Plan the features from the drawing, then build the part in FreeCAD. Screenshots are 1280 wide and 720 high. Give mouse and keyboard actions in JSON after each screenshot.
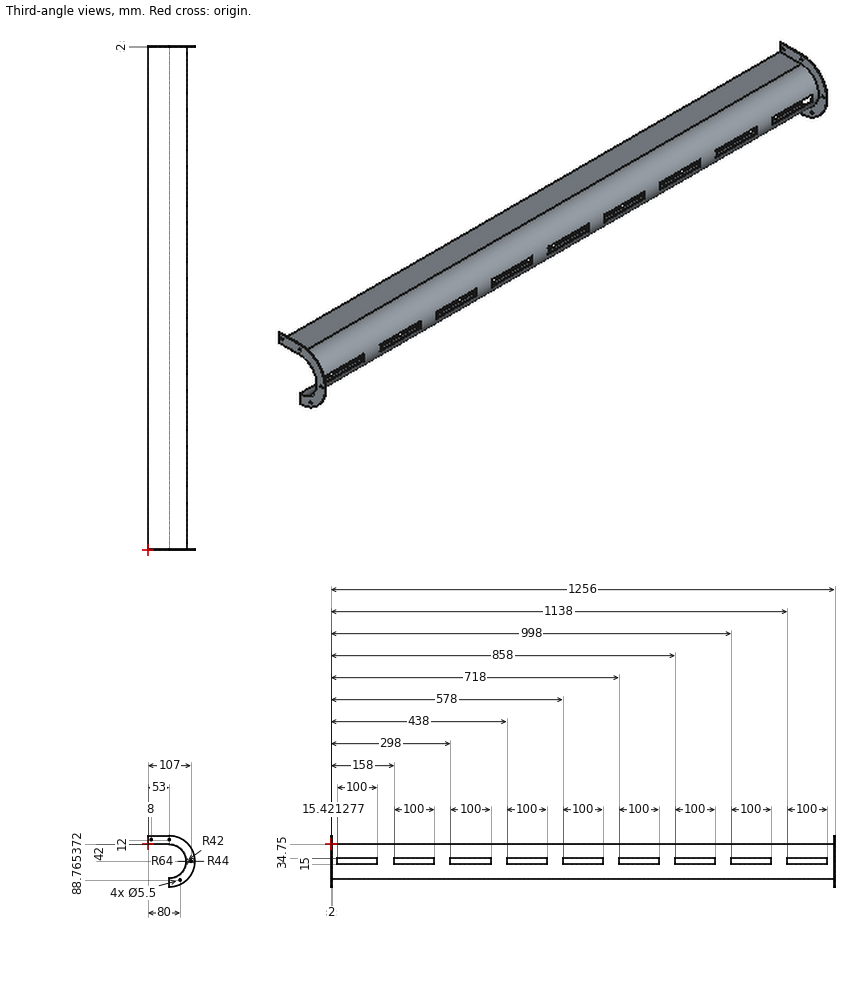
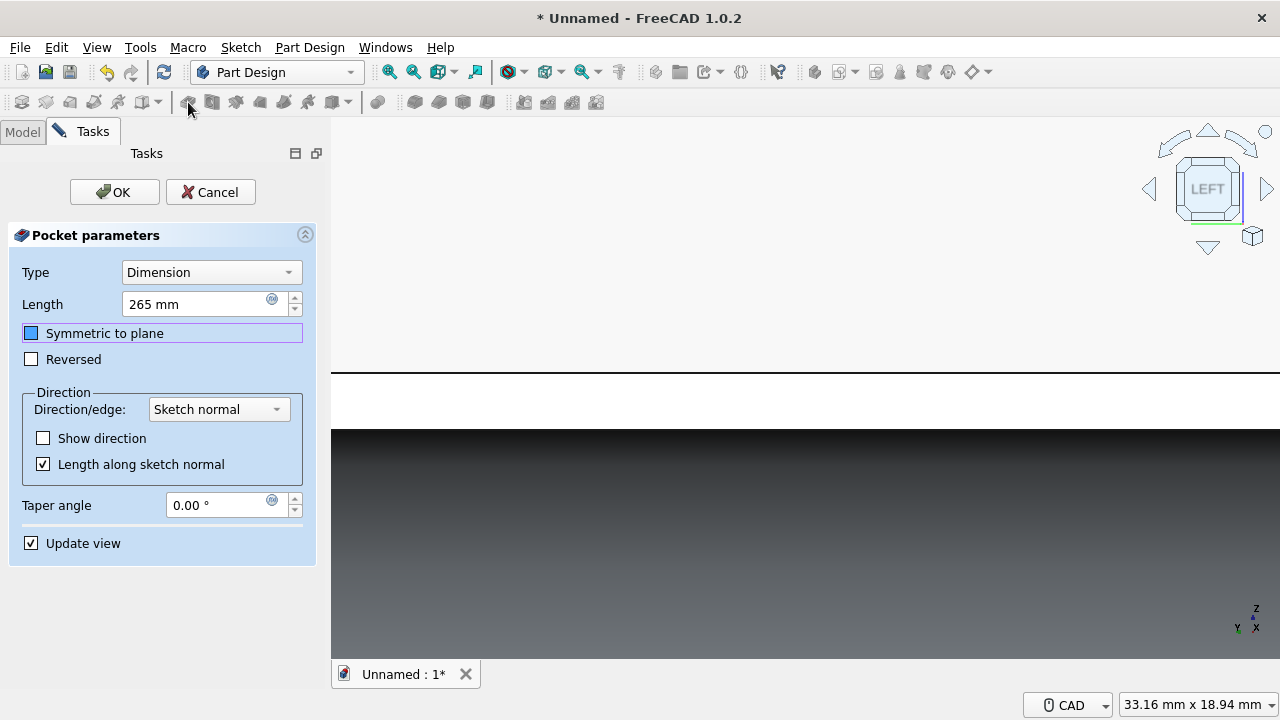
{"action": "left_click", "coordinate": [115, 192]}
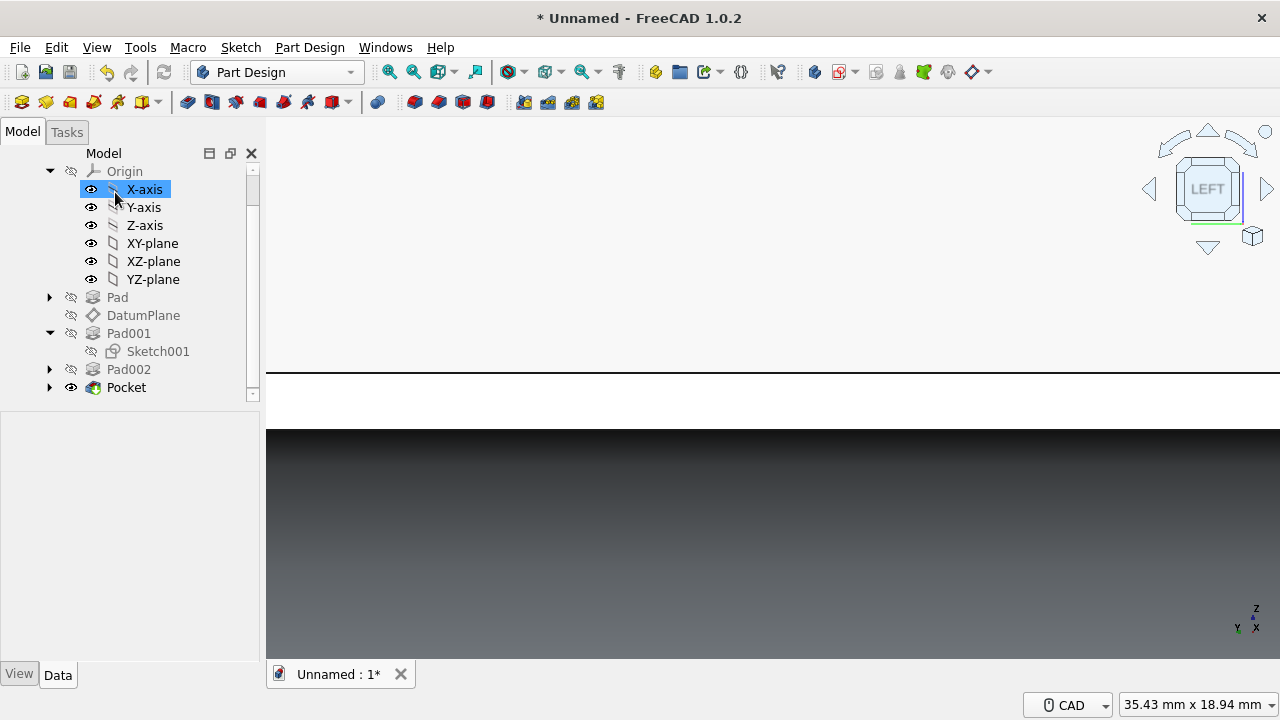
{"action": "left_click", "coordinate": [390, 72]}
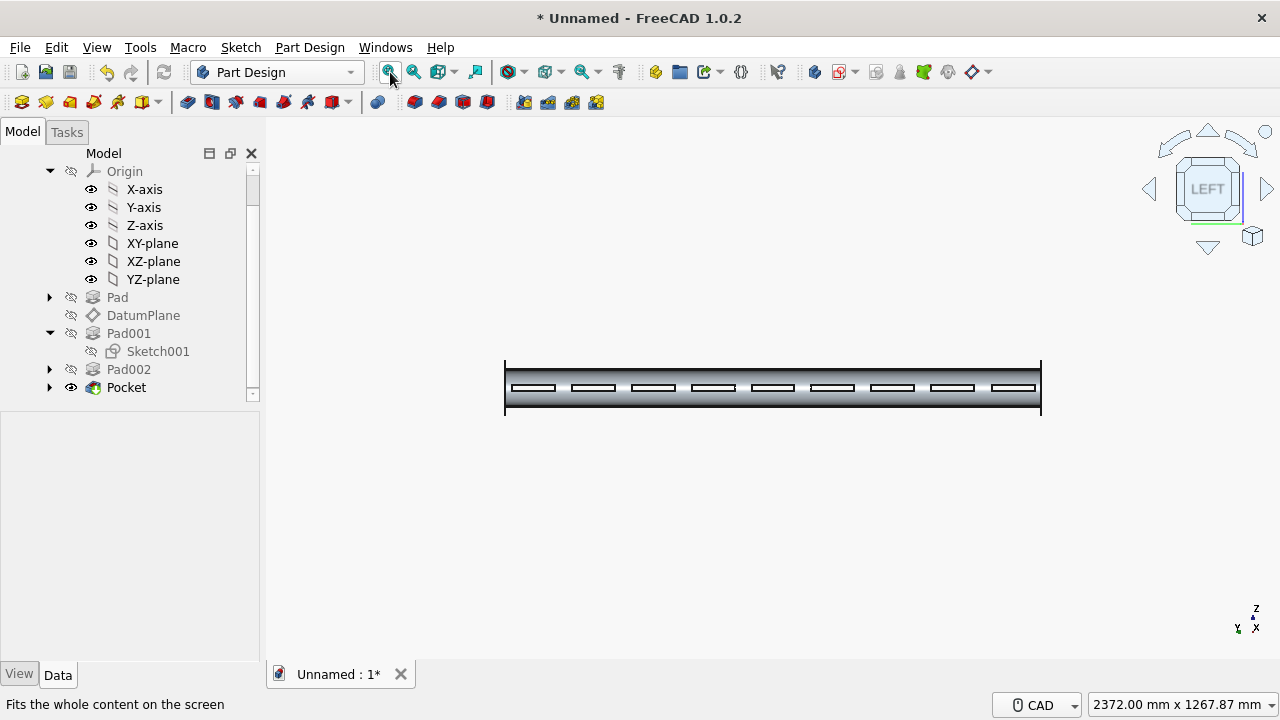
{"action": "key", "text": "4"}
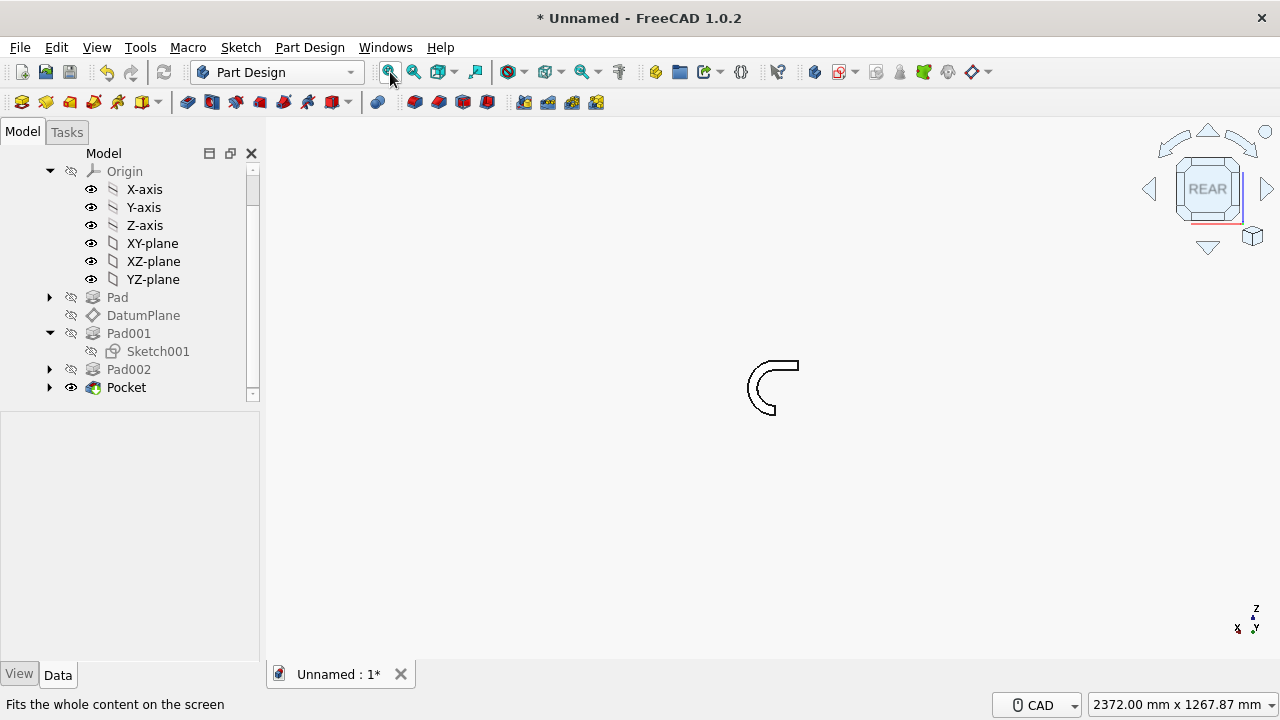
{"action": "left_click", "coordinate": [390, 72]}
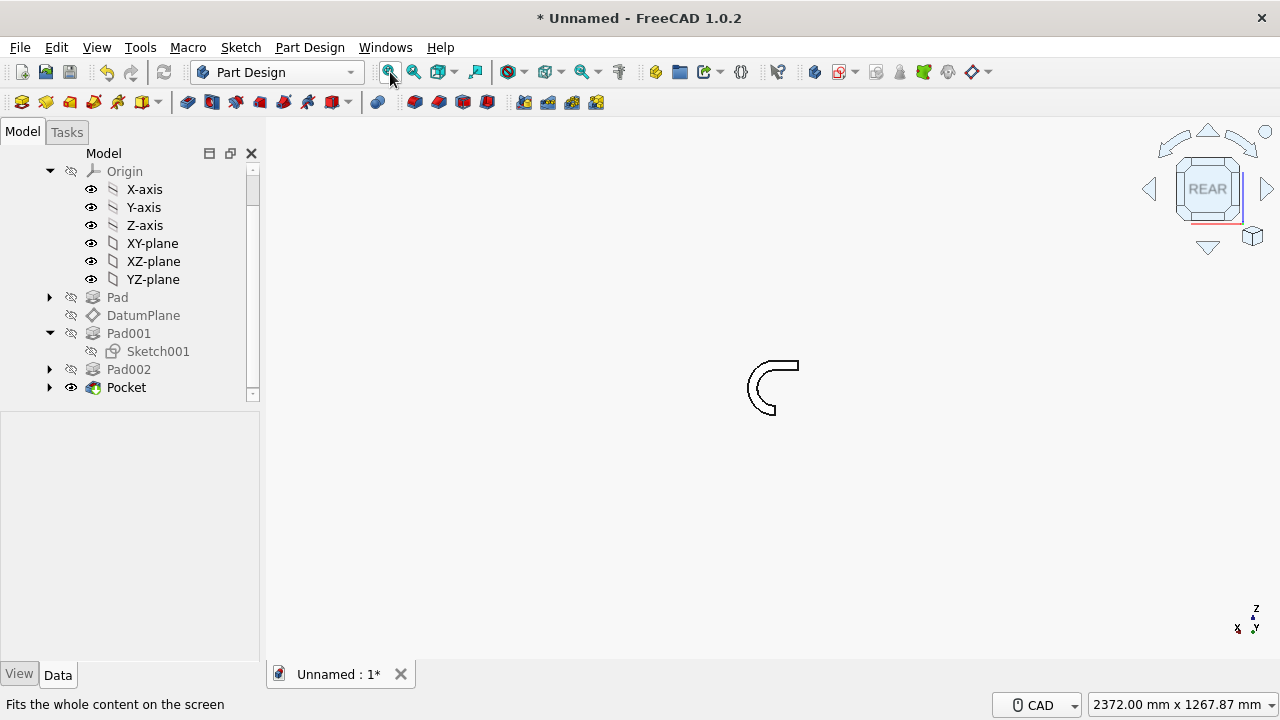
{"action": "scroll", "coordinate": [759, 403], "scroll_direction": "up", "scroll_amount": 5}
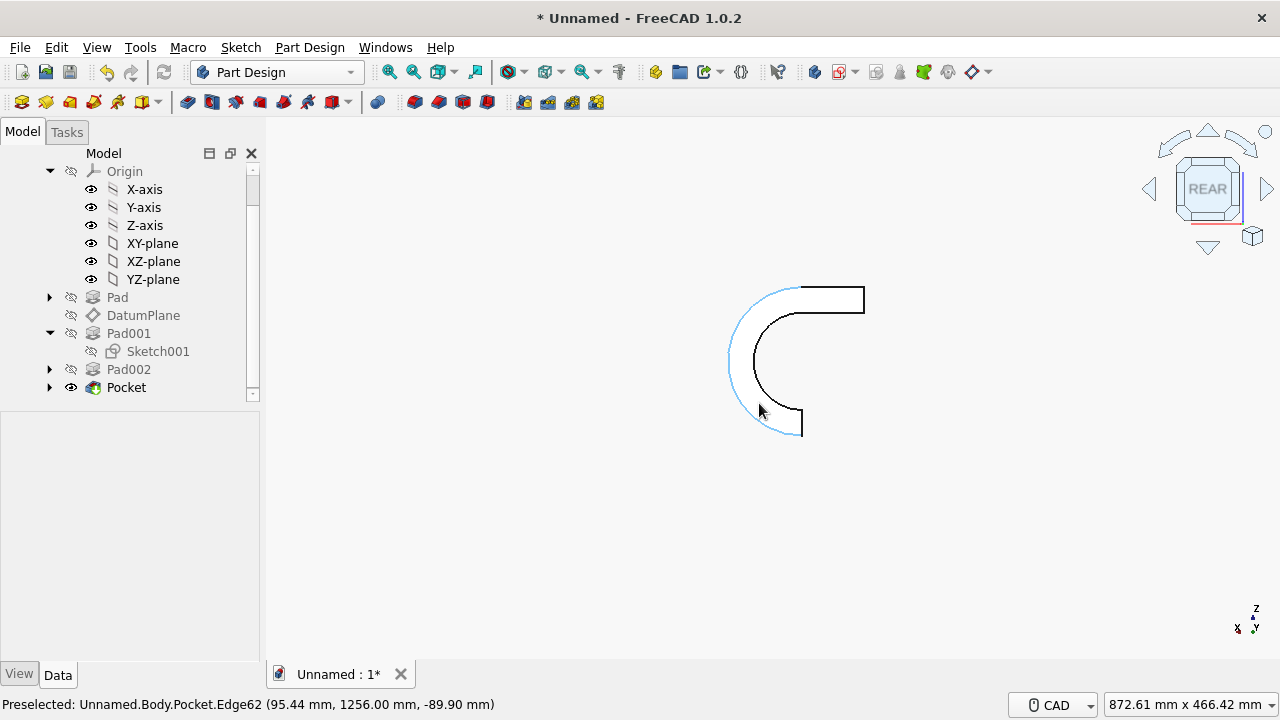
{"action": "left_click", "coordinate": [757, 403]}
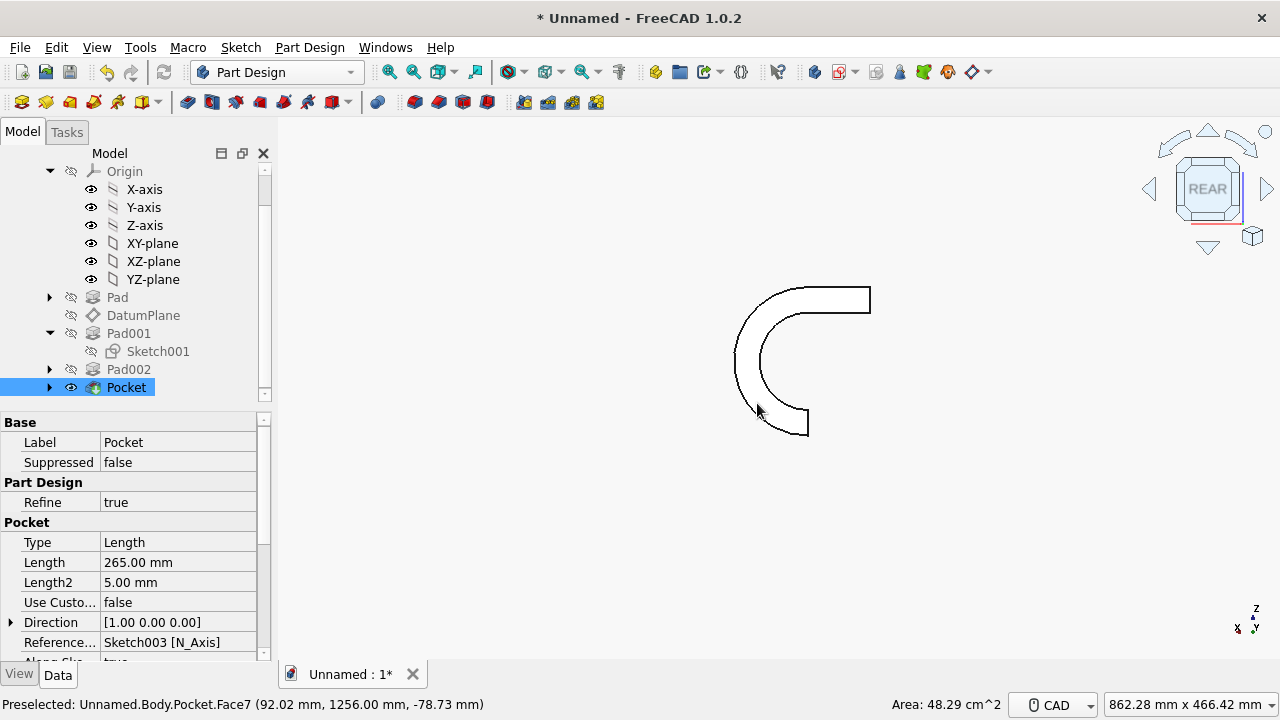
{"action": "left_click", "coordinate": [840, 72]}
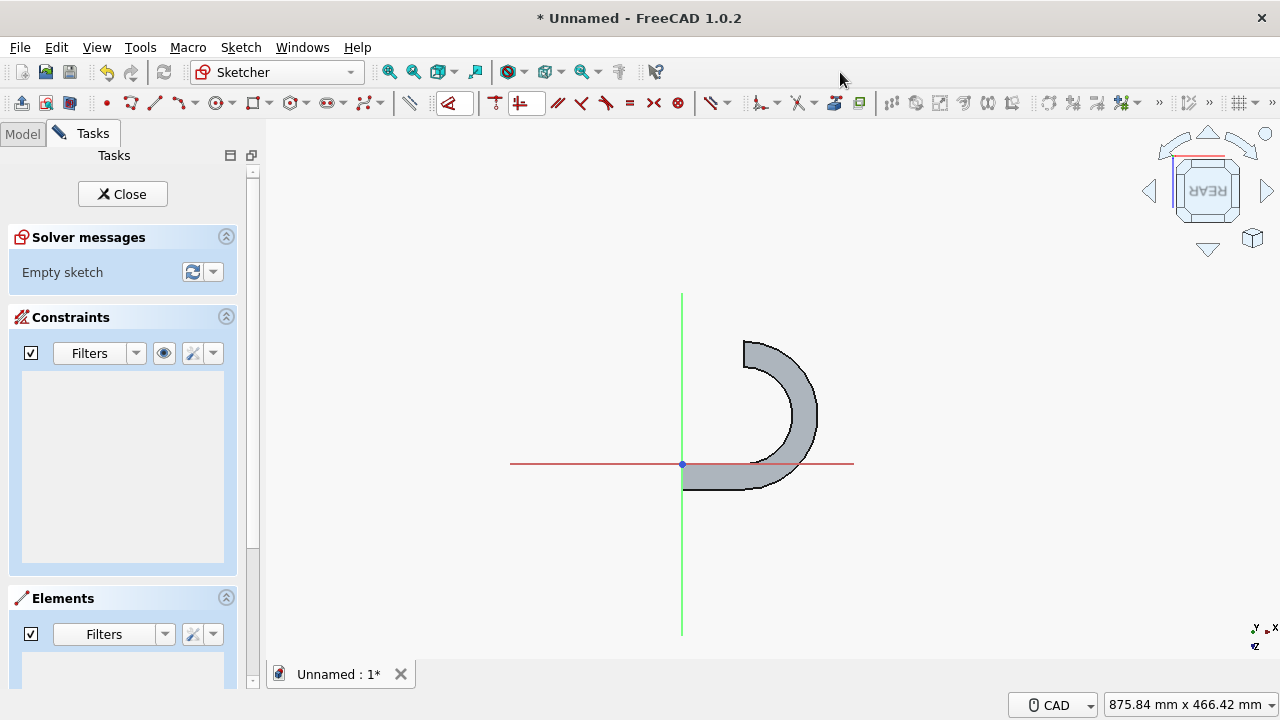
{"action": "scroll", "coordinate": [770, 438], "scroll_direction": "up", "scroll_amount": 5}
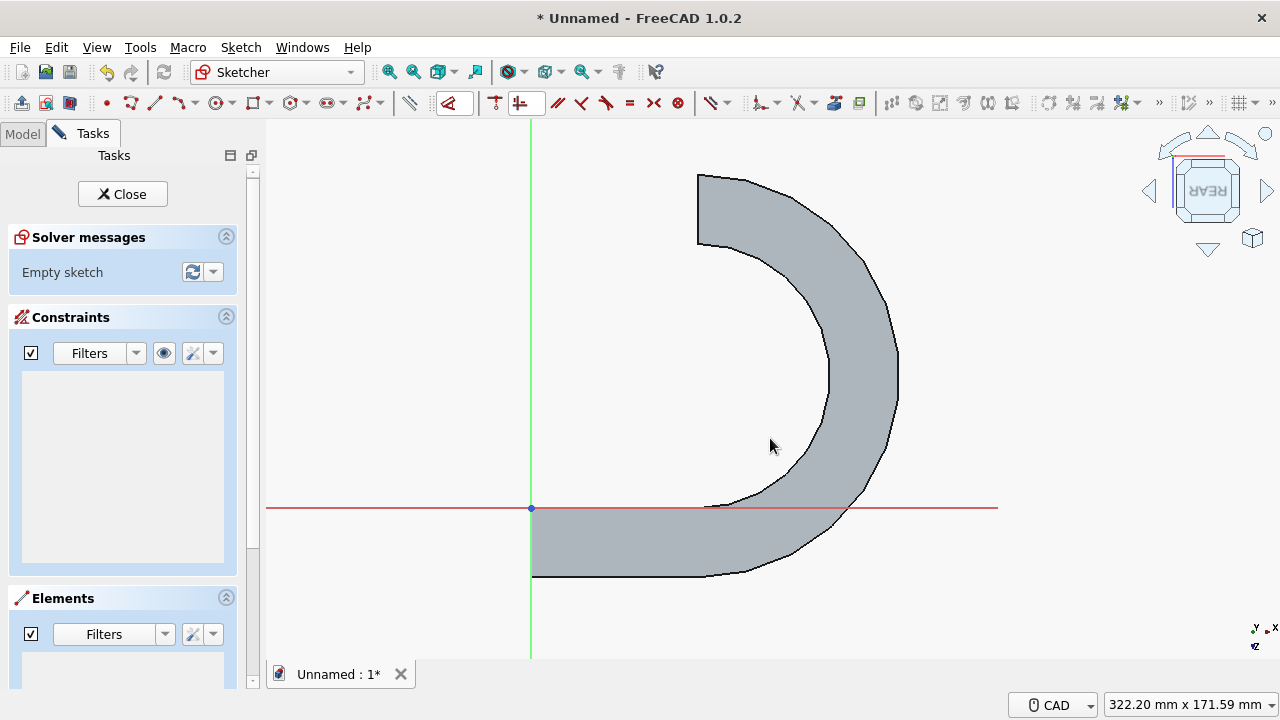
{"action": "key", "text": "g c"}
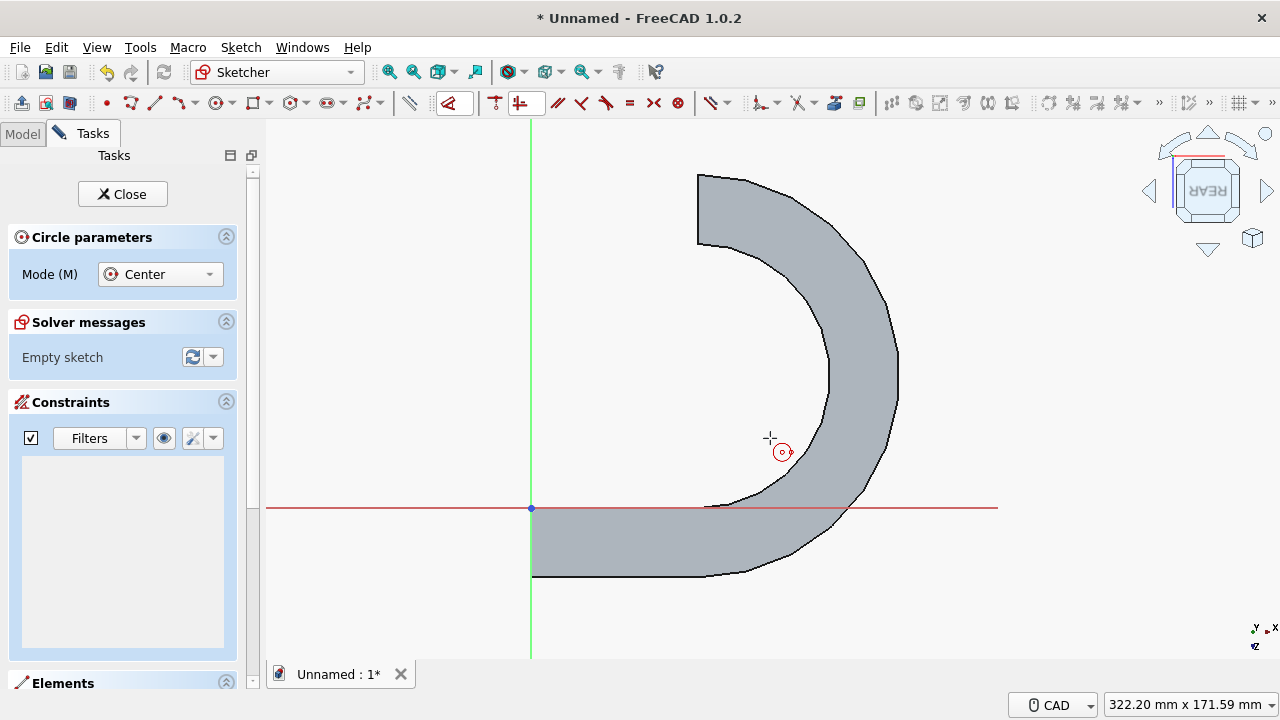
{"action": "scroll", "coordinate": [783, 229], "scroll_direction": "up", "scroll_amount": 5}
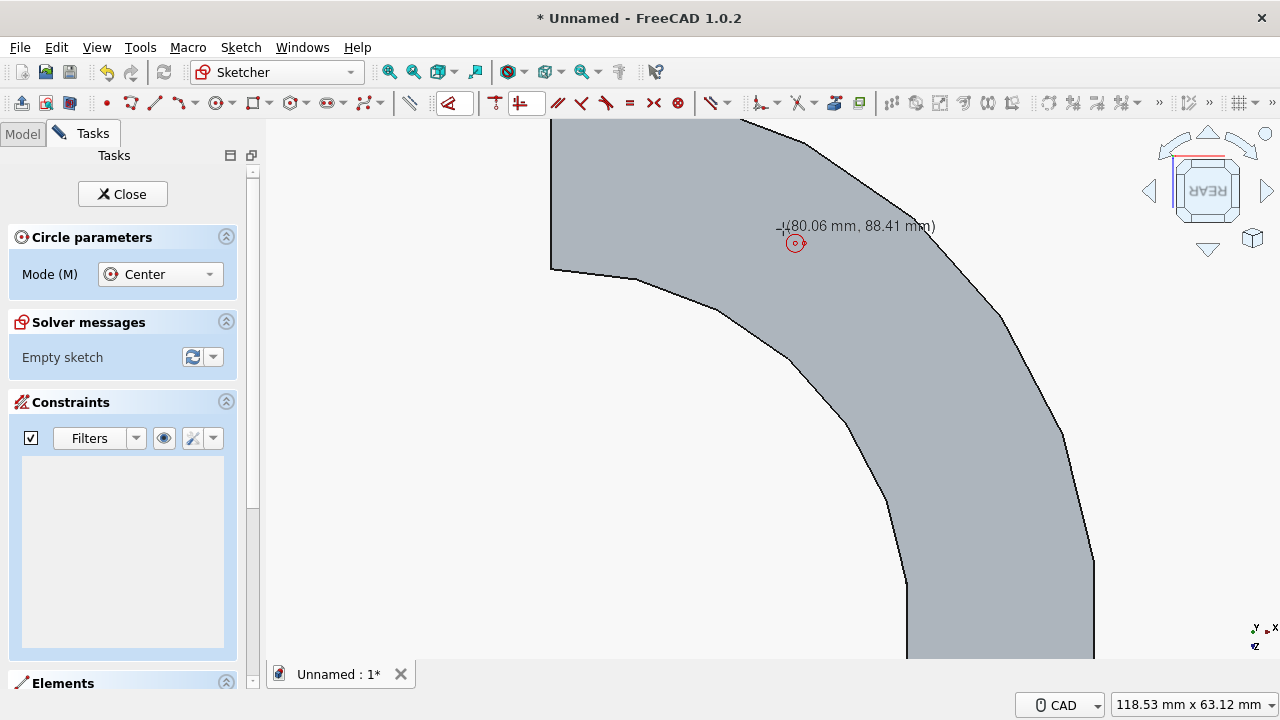
{"action": "left_click", "coordinate": [782, 228]}
{"action": "left_click", "coordinate": [798, 212]}